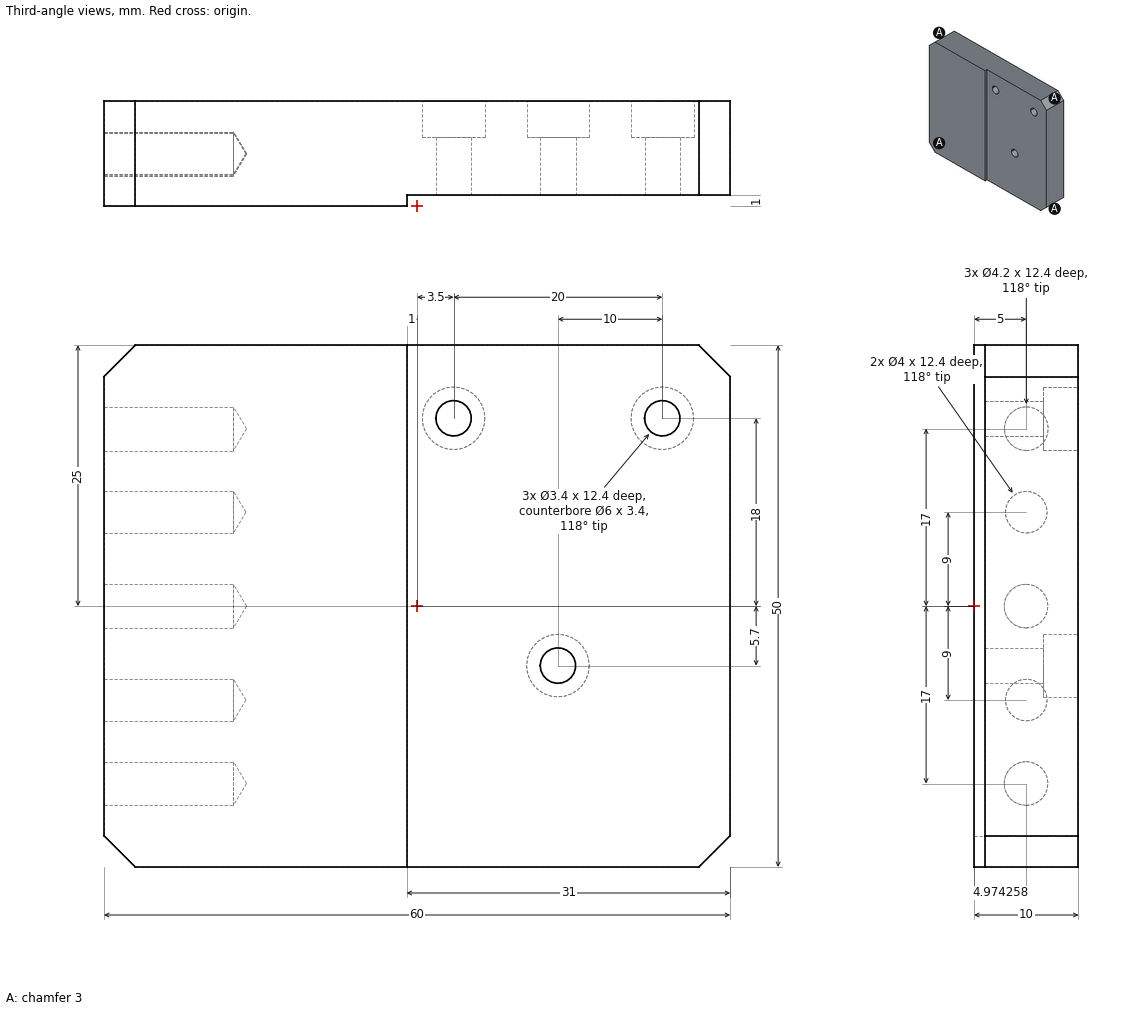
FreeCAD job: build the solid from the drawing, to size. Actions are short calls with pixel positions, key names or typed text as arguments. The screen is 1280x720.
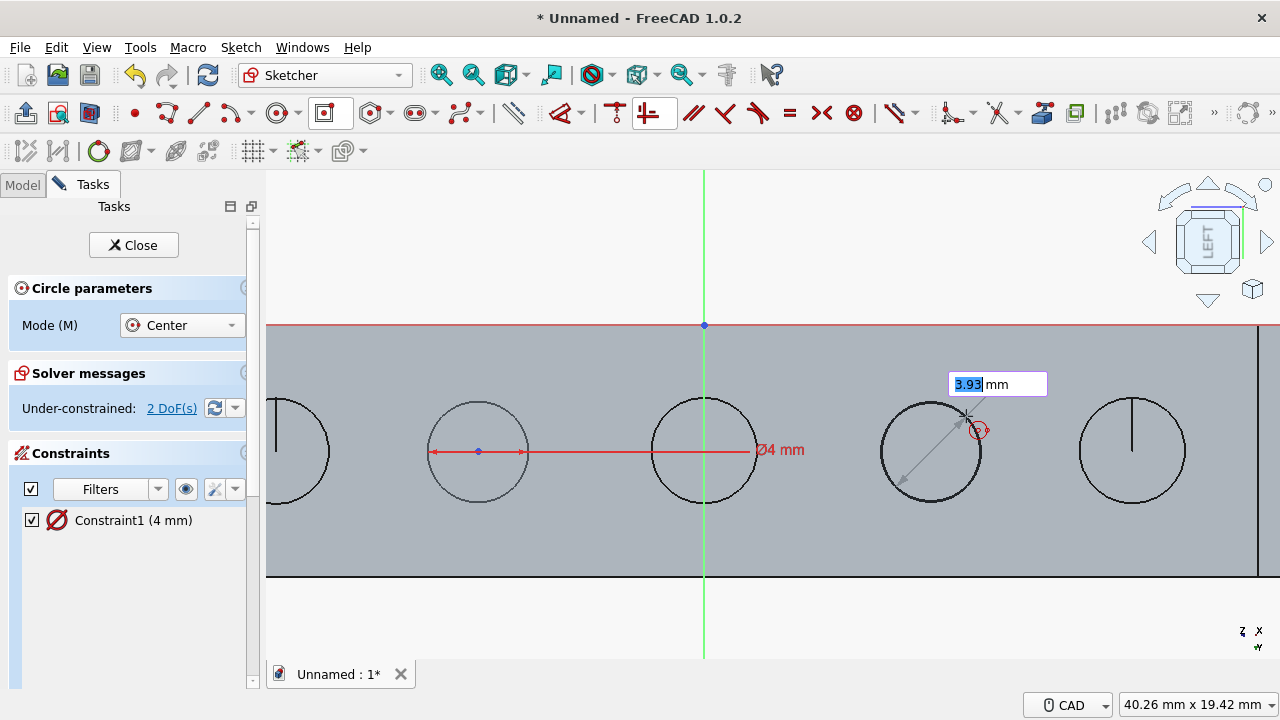
text(4)
key(Return)
key(Escape)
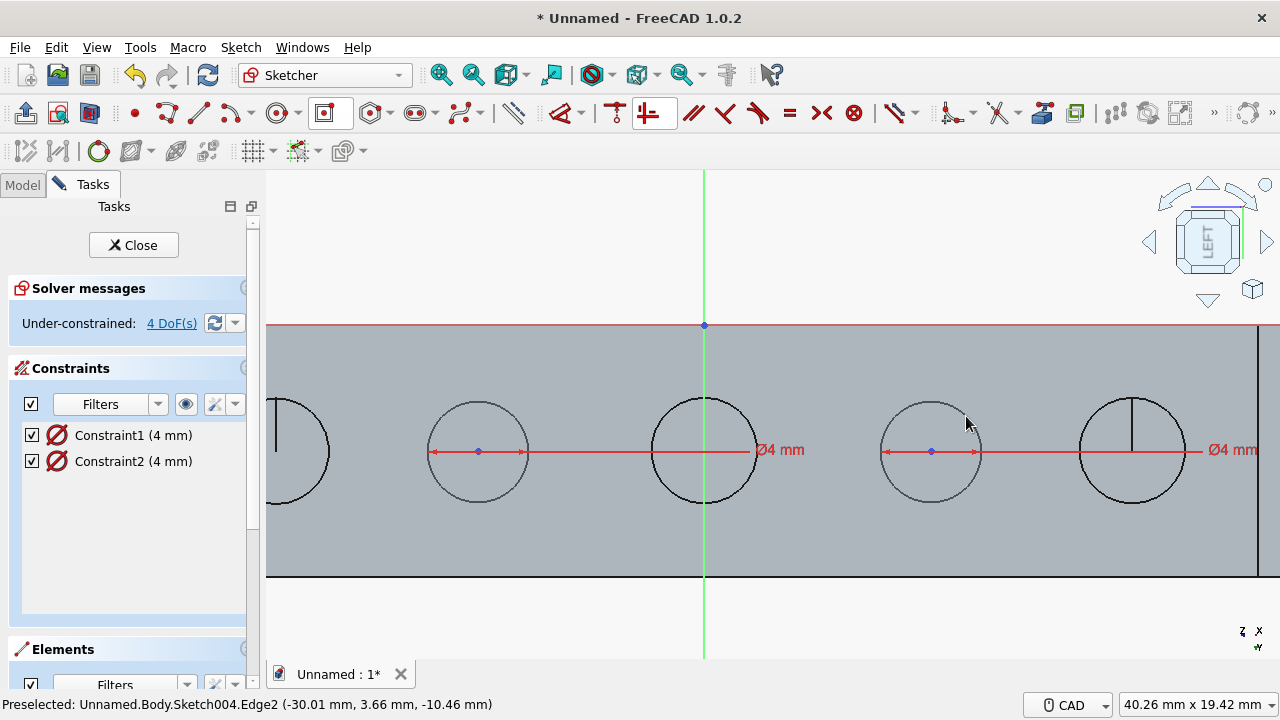
click(478, 452)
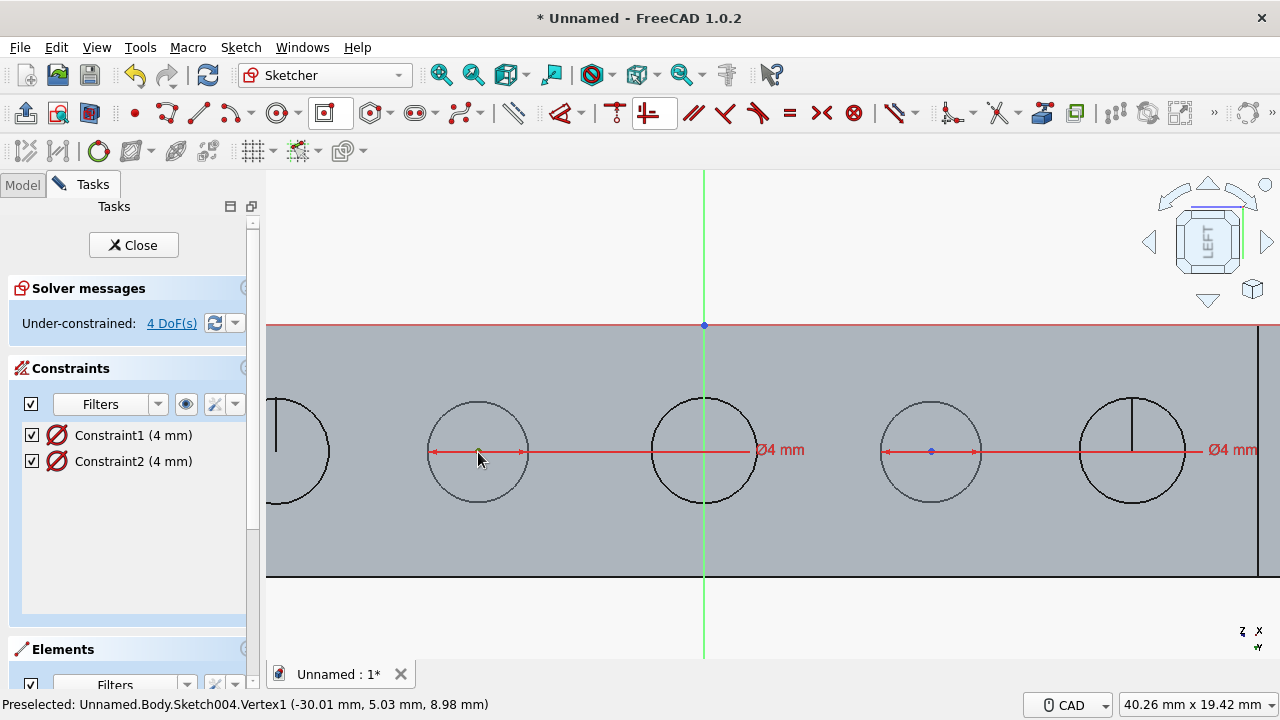
click(931, 452)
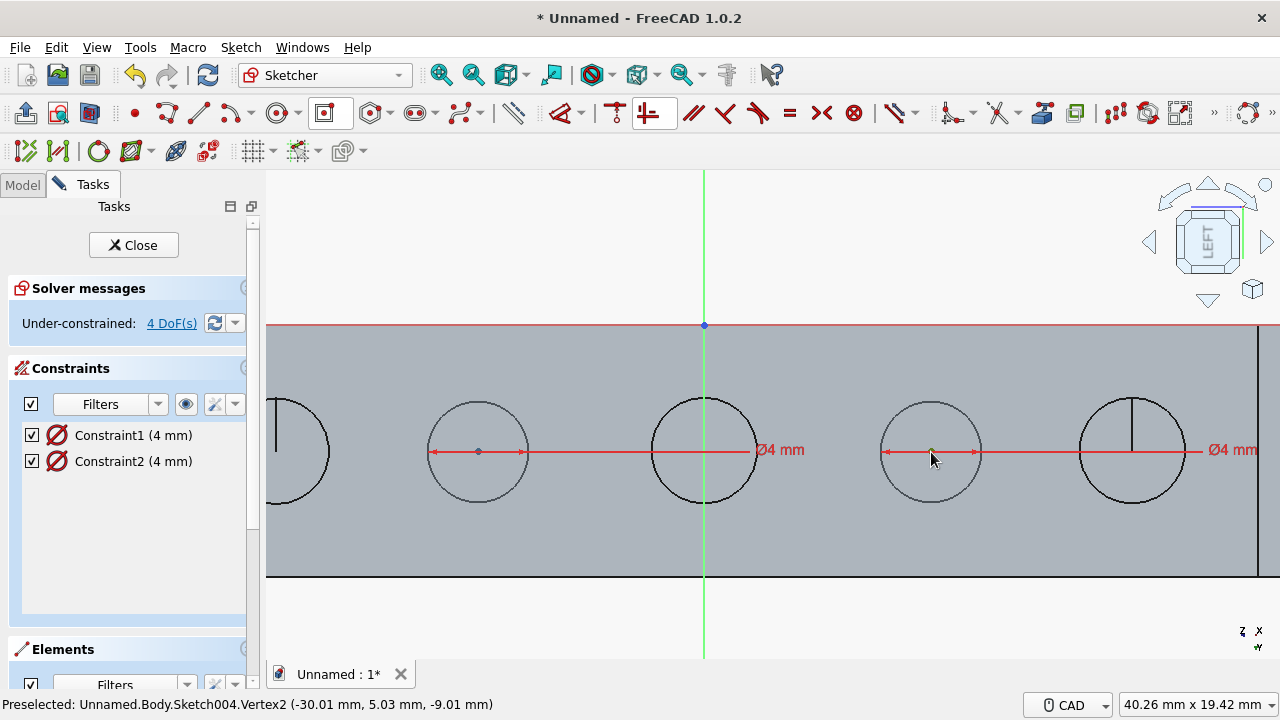
click(672, 114)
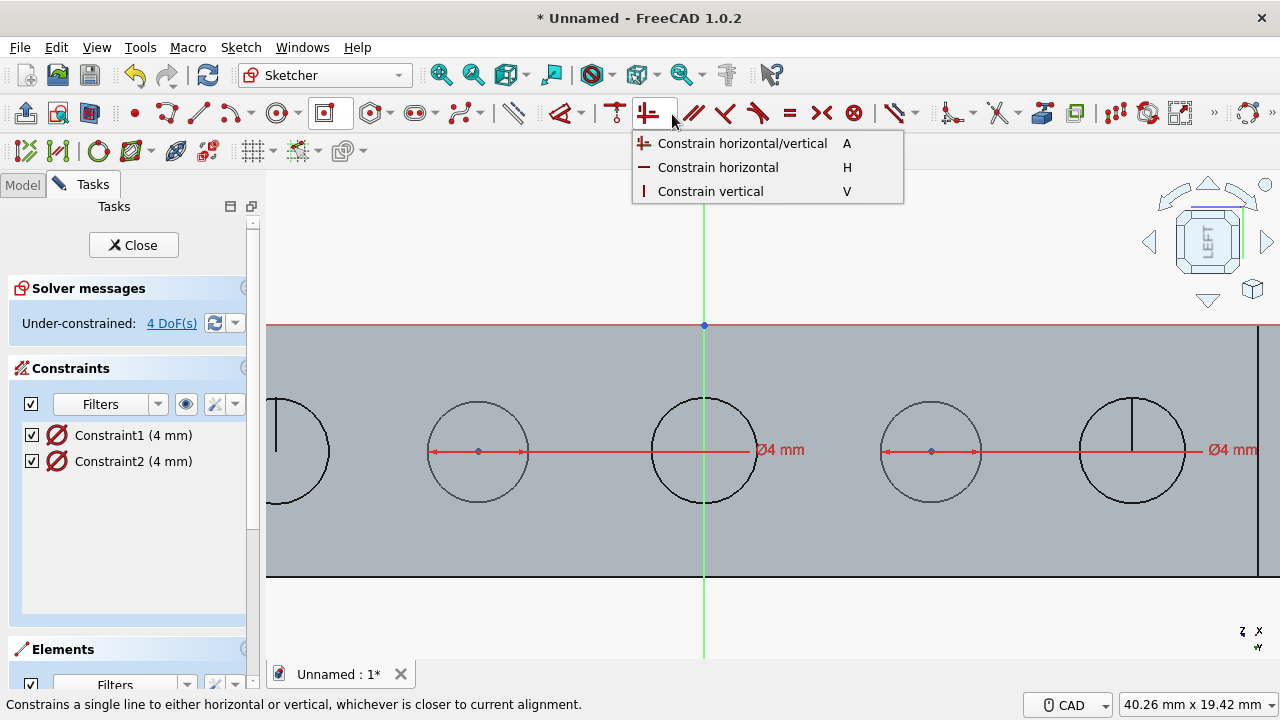
click(768, 167)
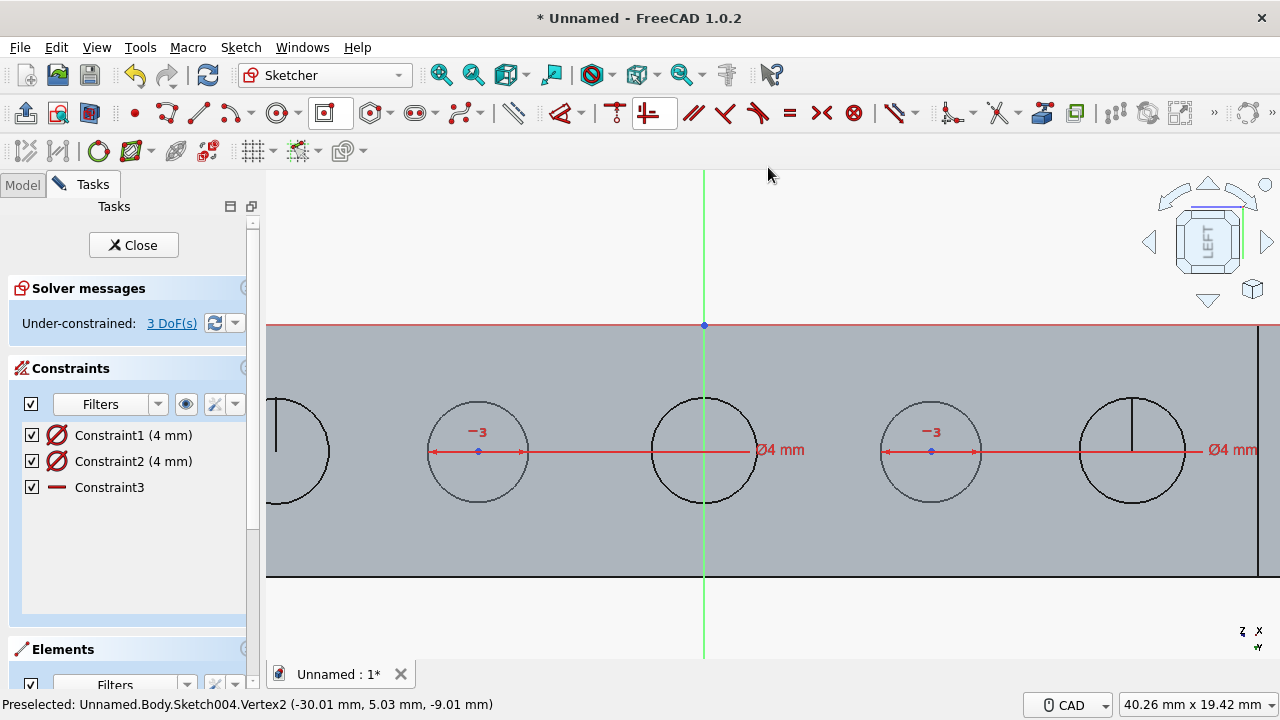
click(560, 114)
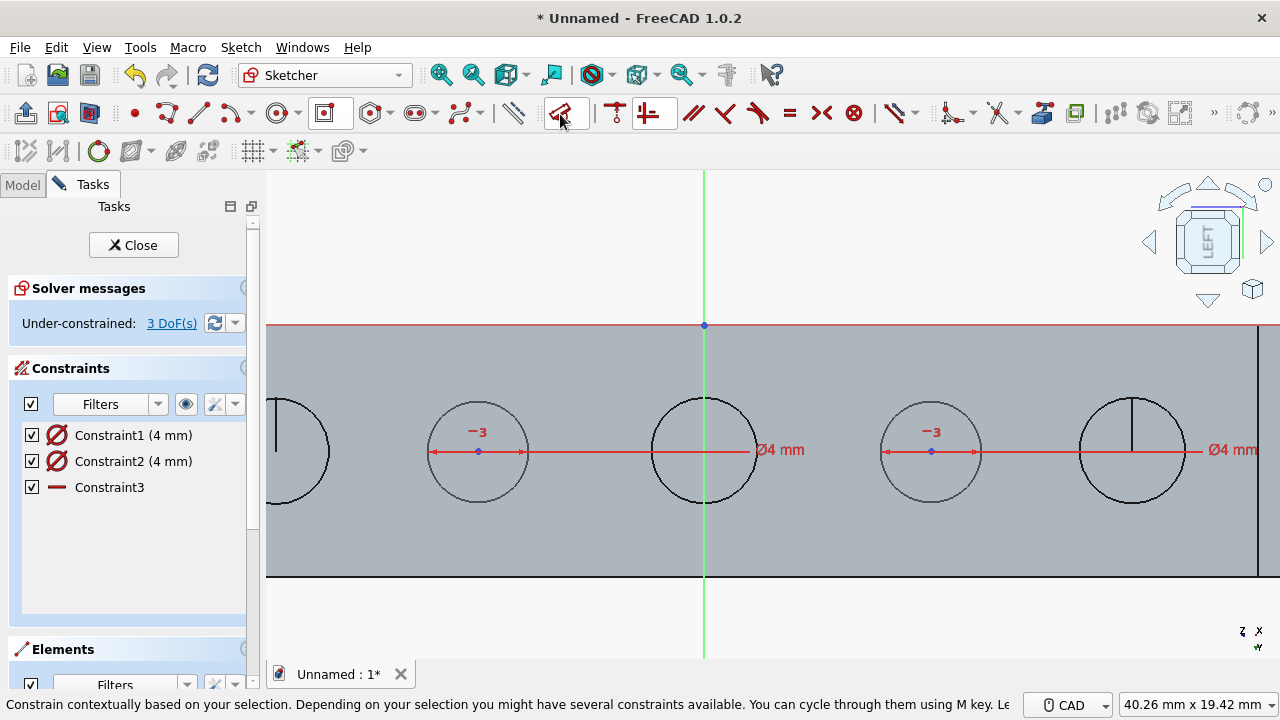
click(478, 452)
click(591, 291)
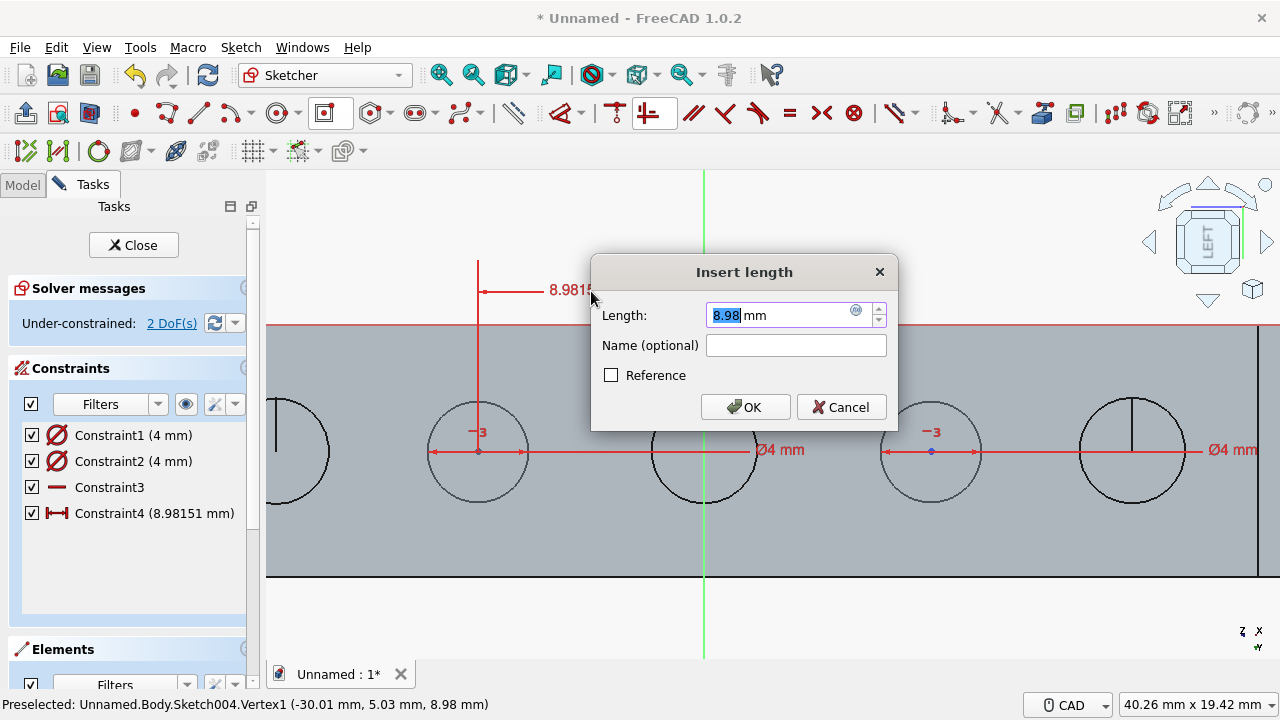
text(9)
key(Return)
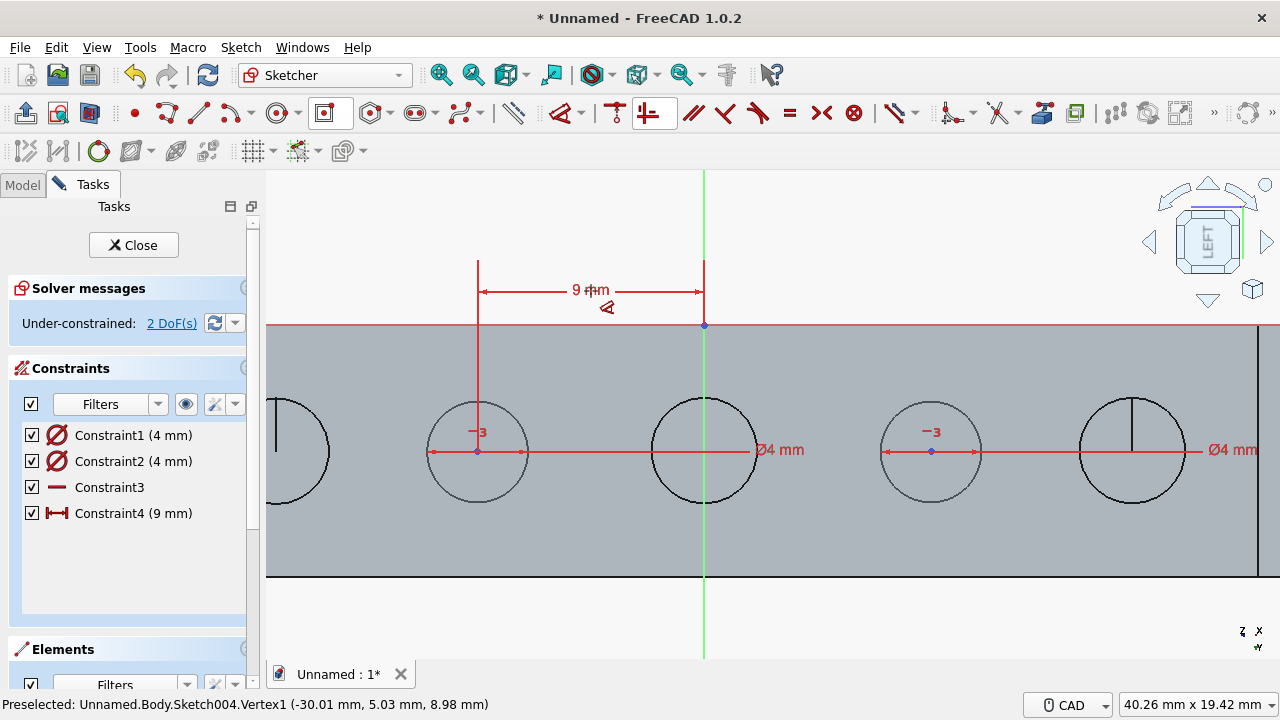
click(478, 452)
click(444, 389)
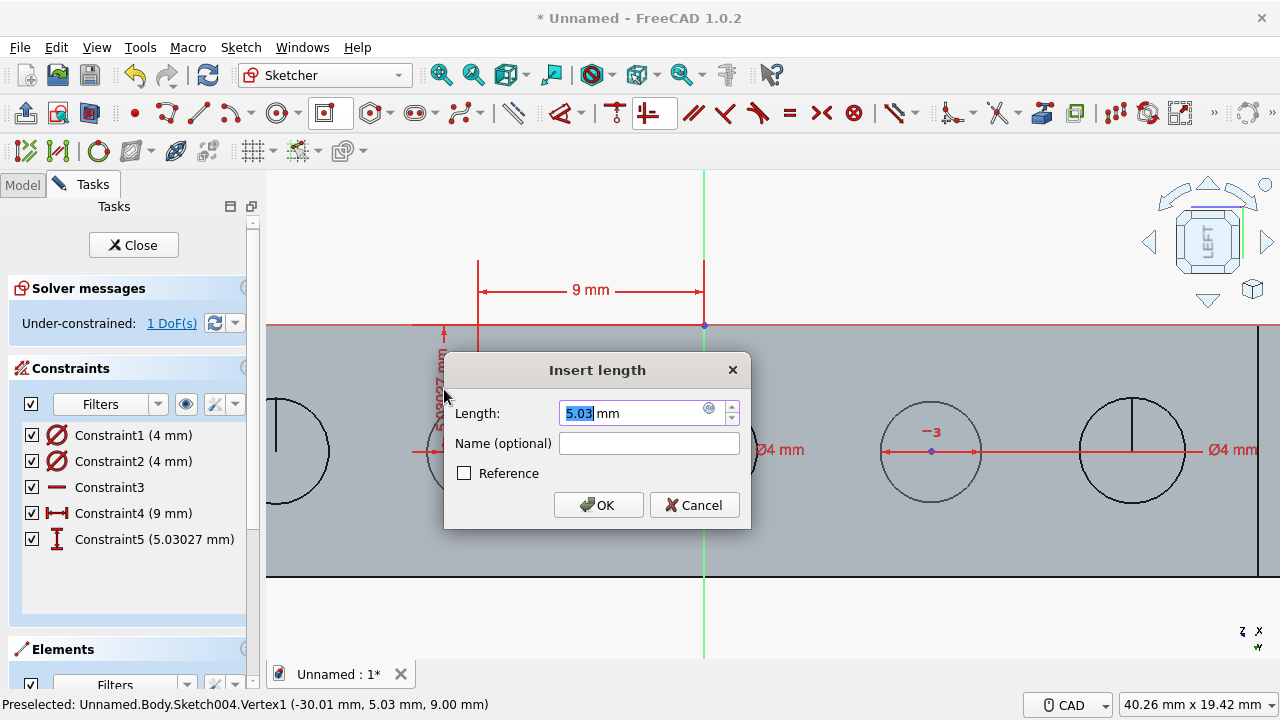
text(5)
key(Return)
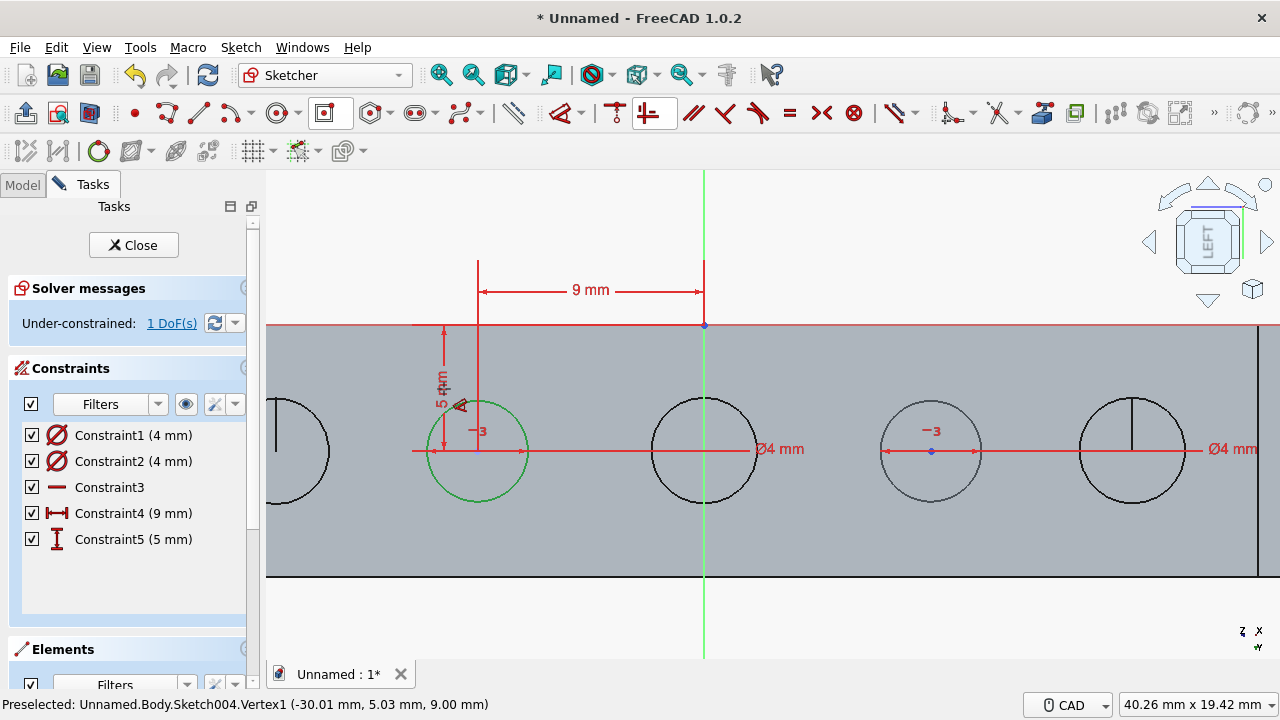
click(931, 451)
click(818, 291)